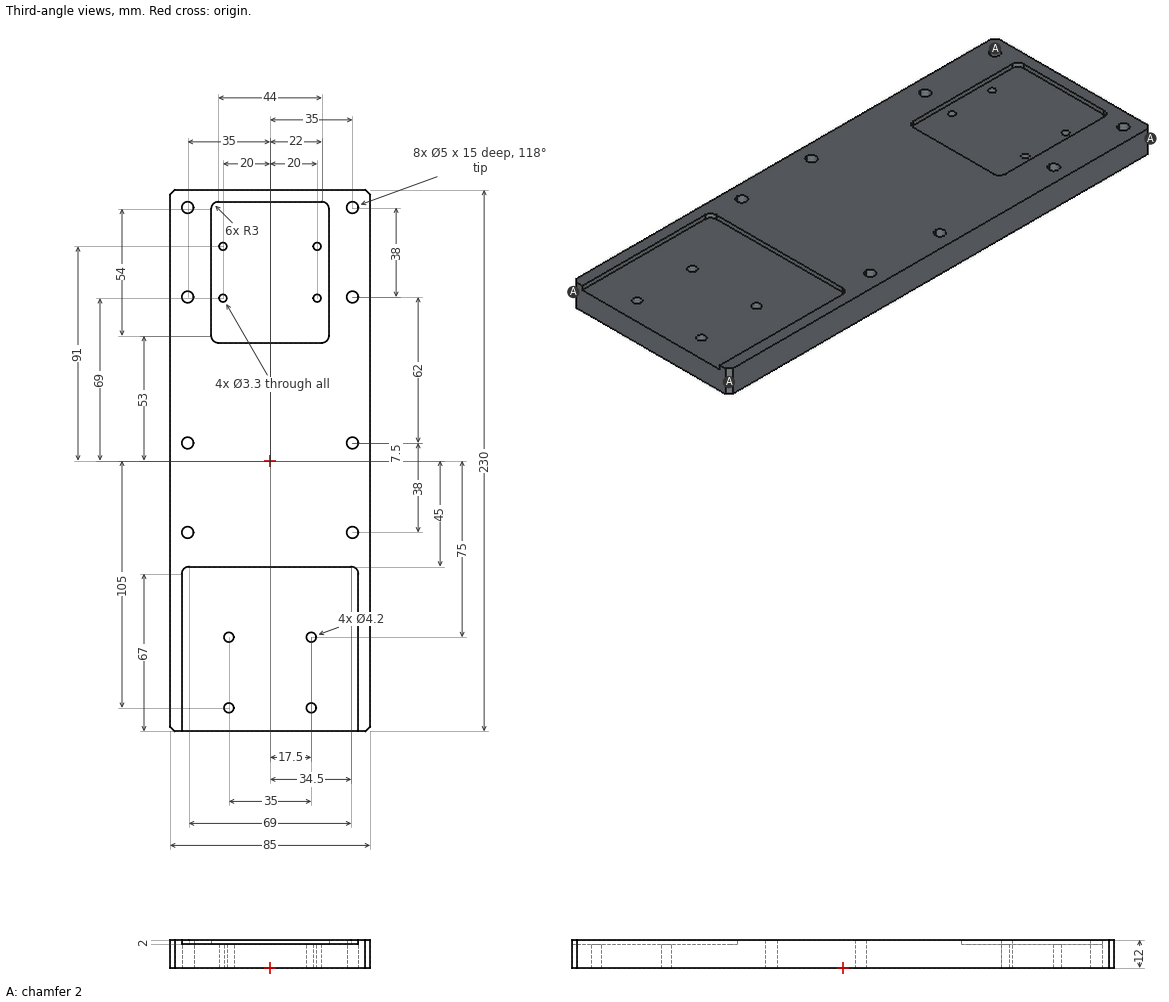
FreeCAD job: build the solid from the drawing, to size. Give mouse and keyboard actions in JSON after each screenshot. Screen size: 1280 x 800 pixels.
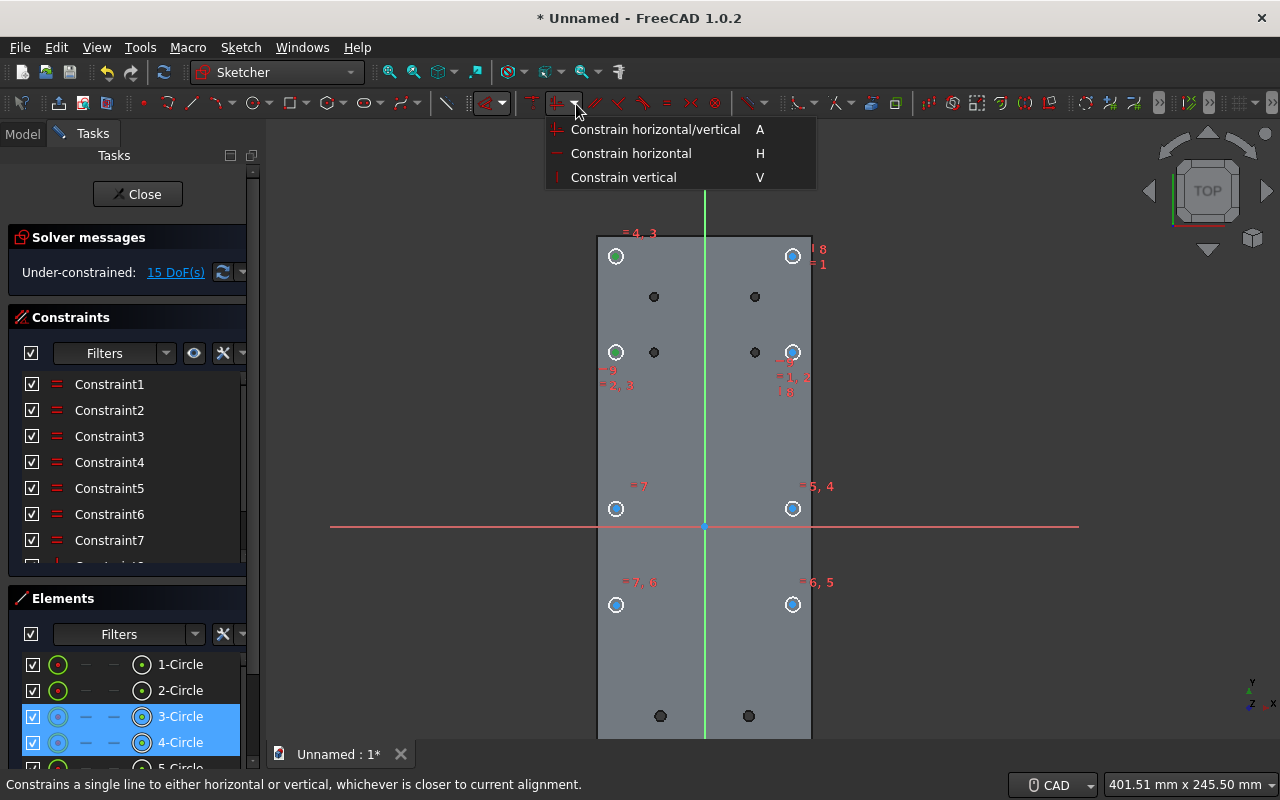
{"action": "left_click", "coordinate": [681, 177]}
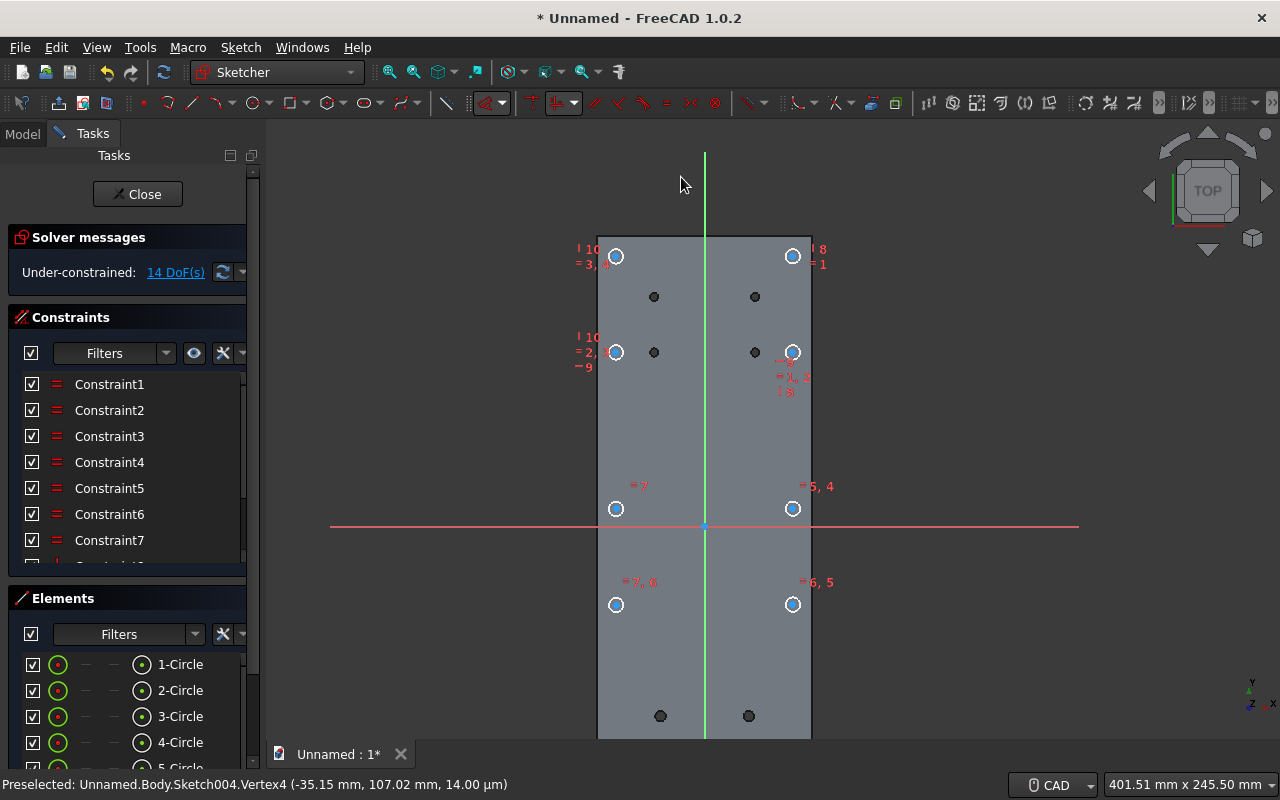
{"action": "left_click", "coordinate": [793, 256]}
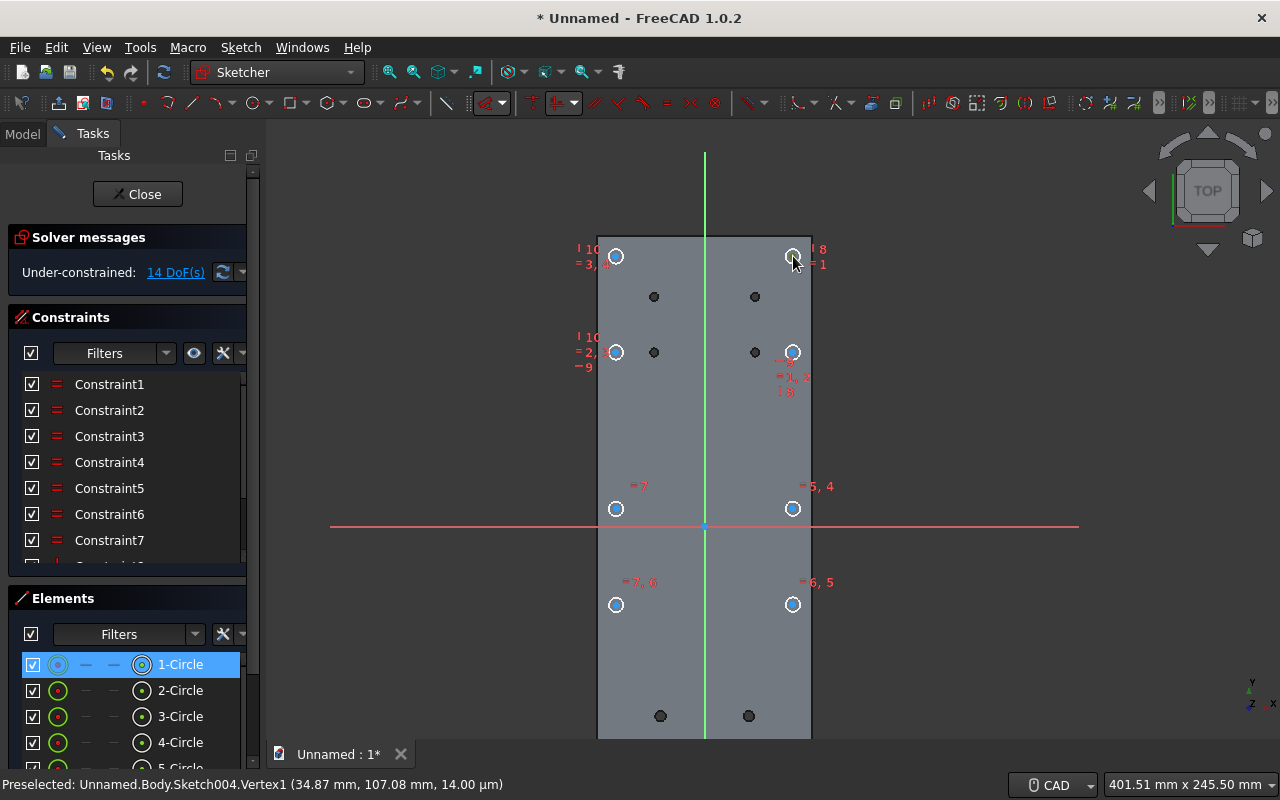
{"action": "left_click", "coordinate": [616, 256]}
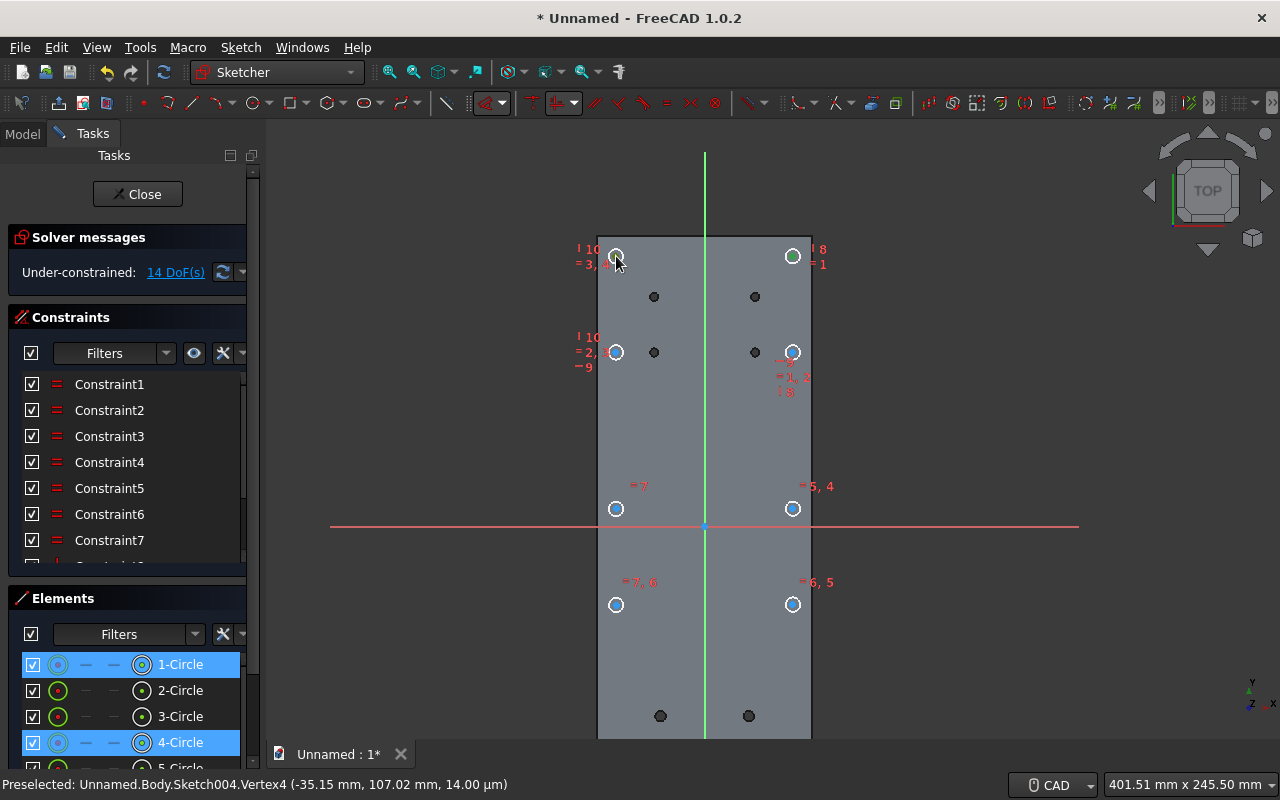
{"action": "key", "text": "h"}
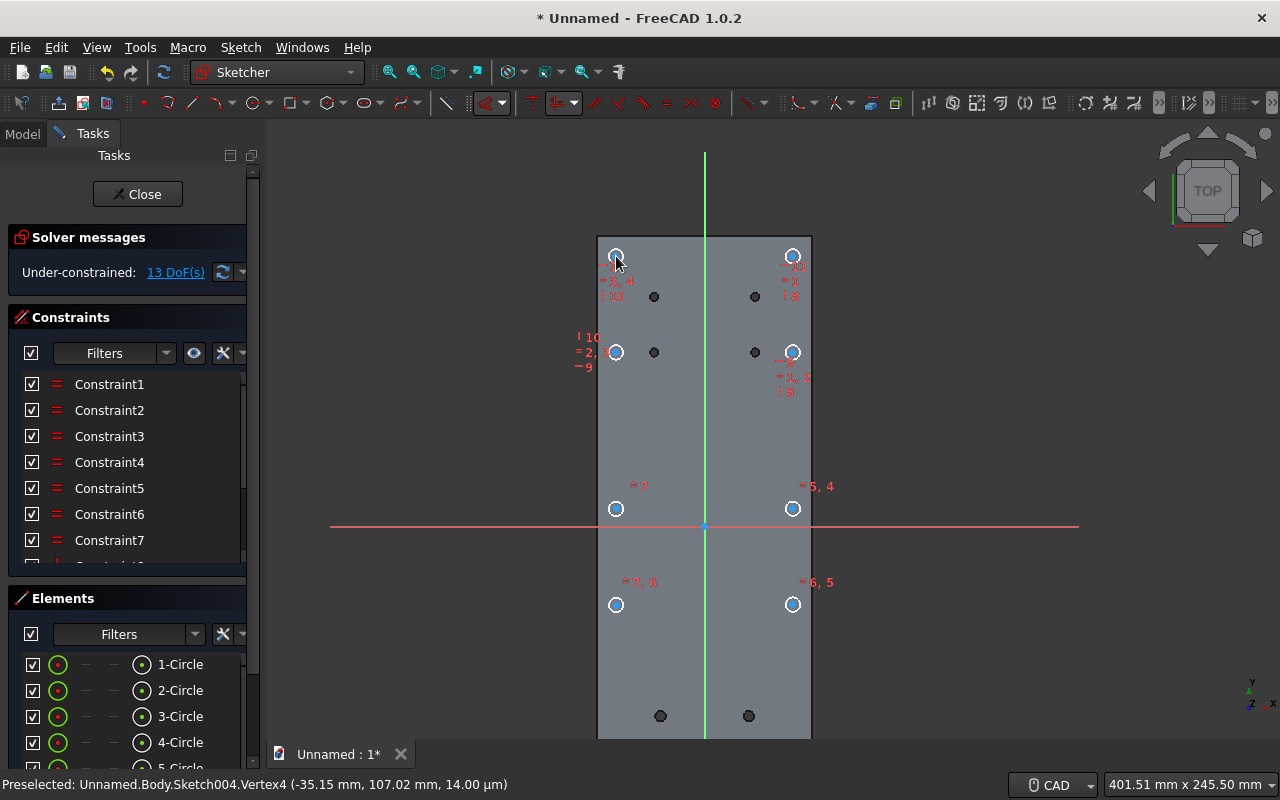
{"action": "left_click", "coordinate": [793, 352]}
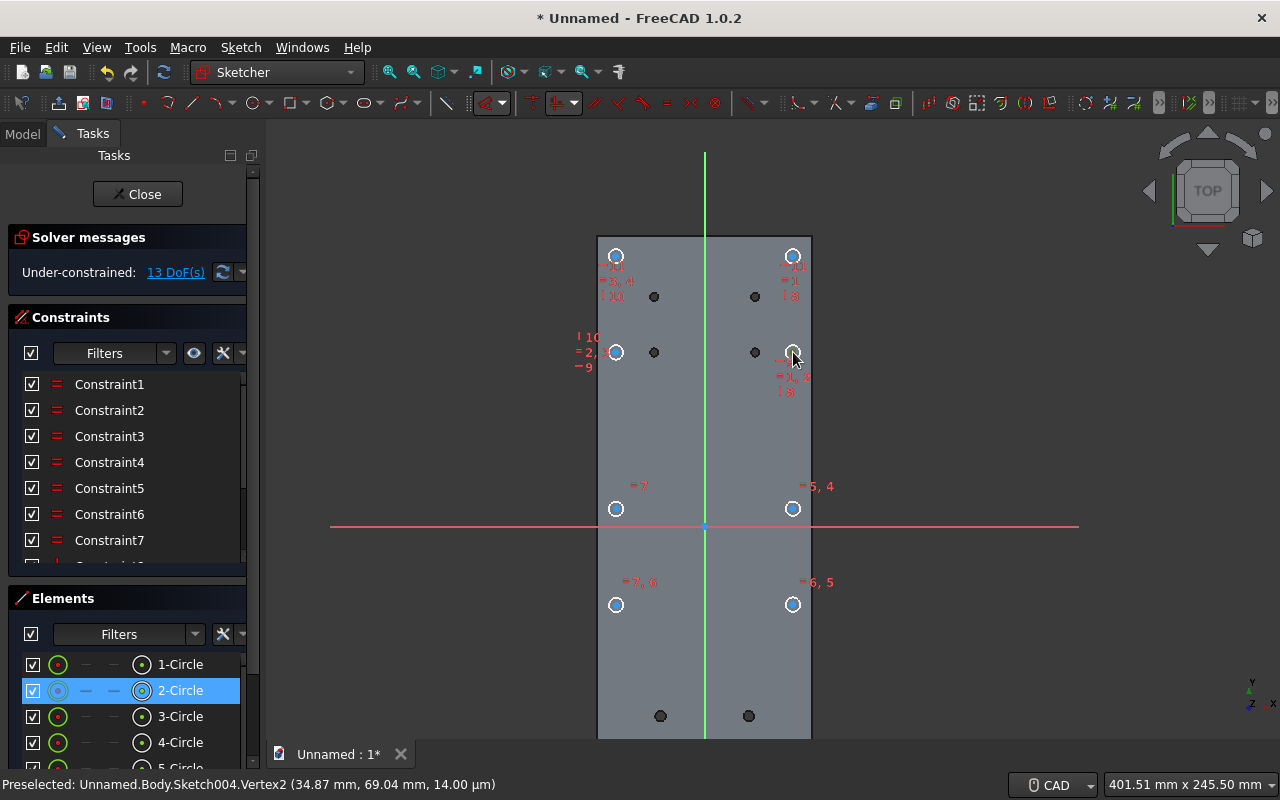
{"action": "left_click", "coordinate": [793, 509]}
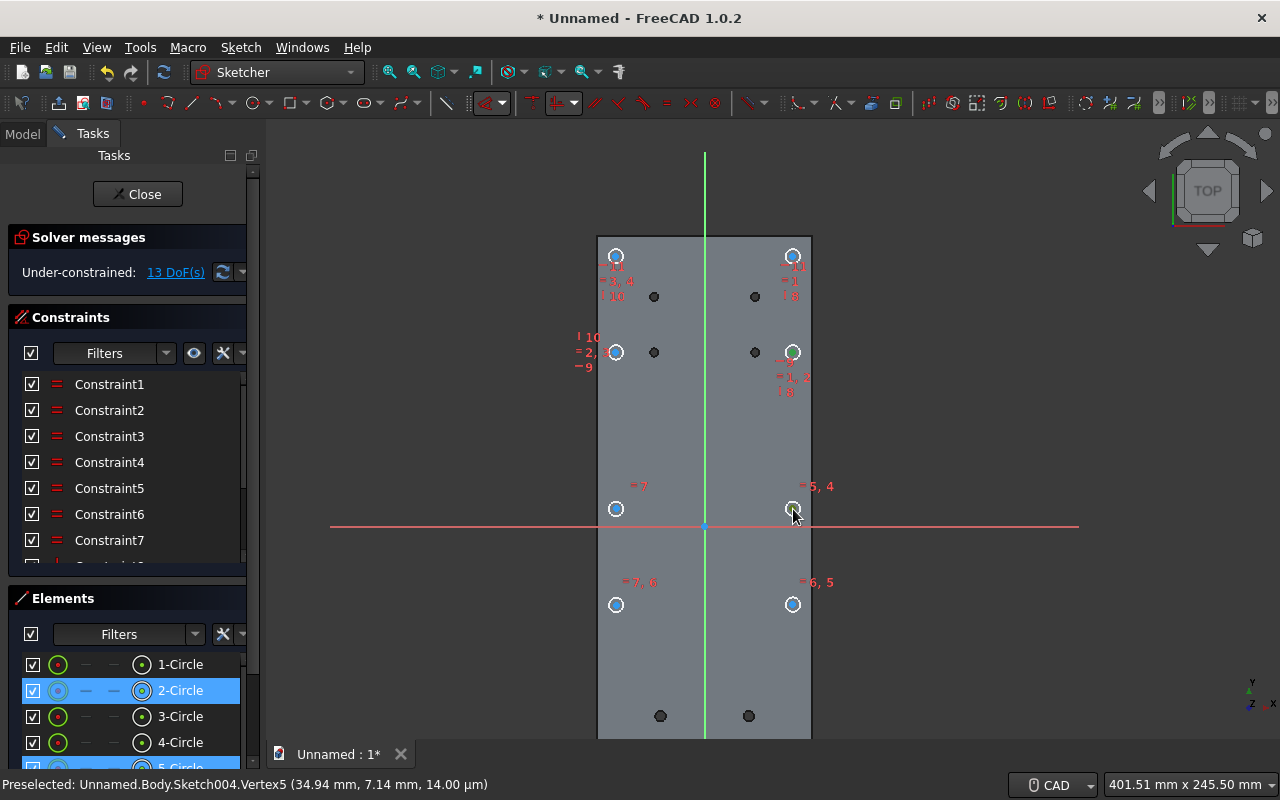
{"action": "key", "text": "v"}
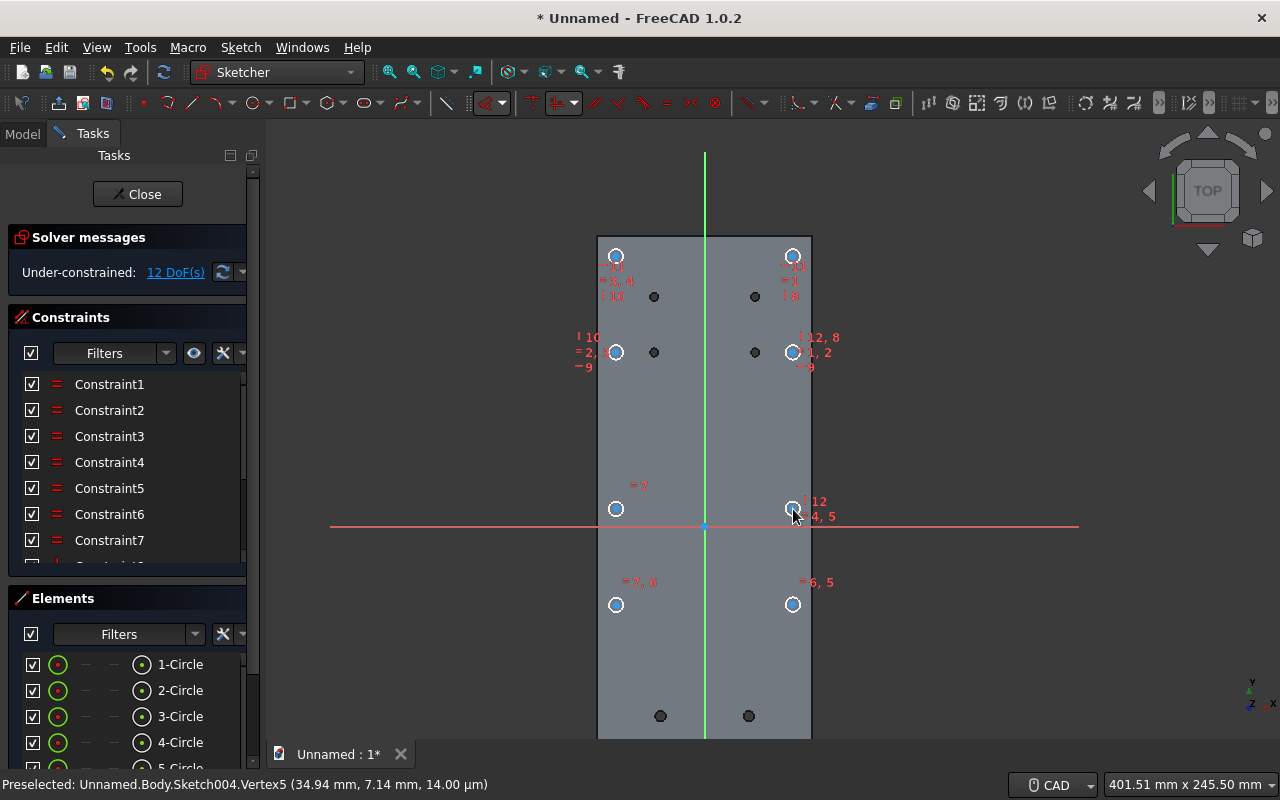
{"action": "left_click", "coordinate": [793, 509]}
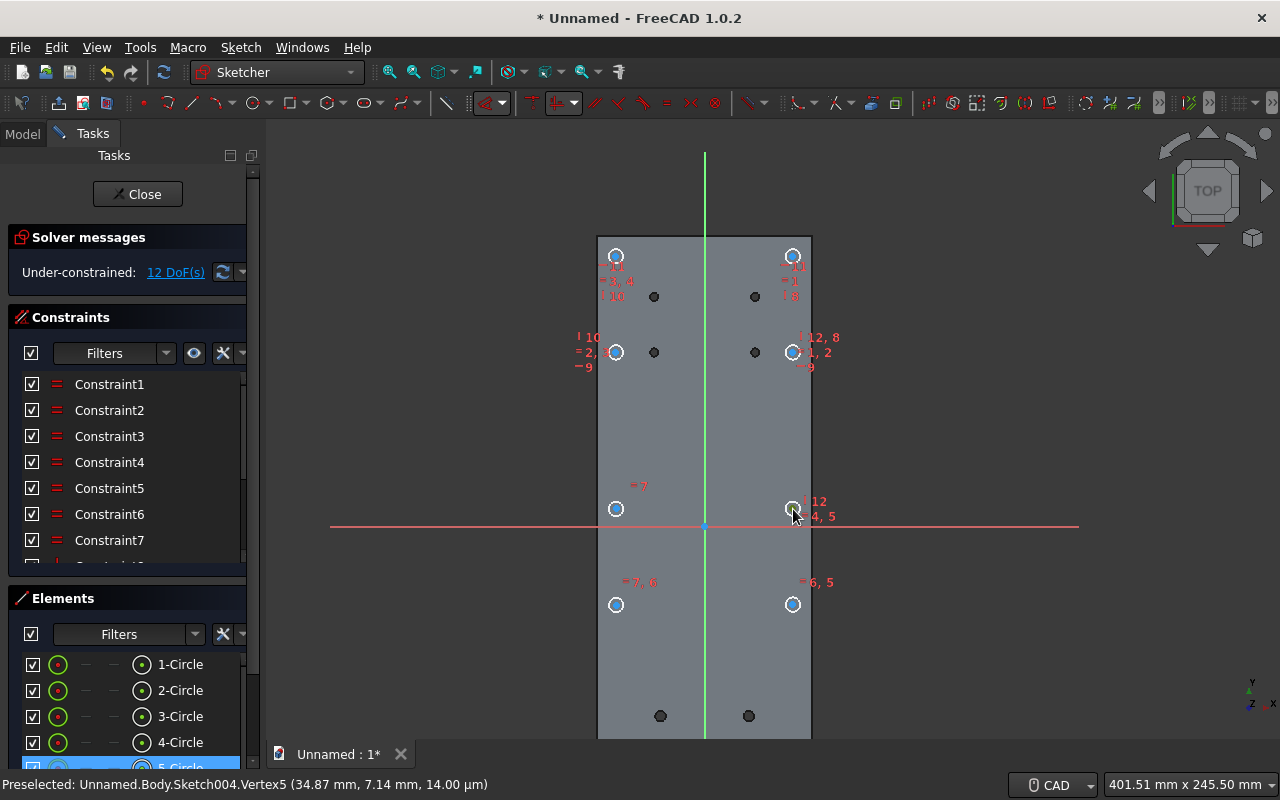
{"action": "left_click", "coordinate": [793, 605]}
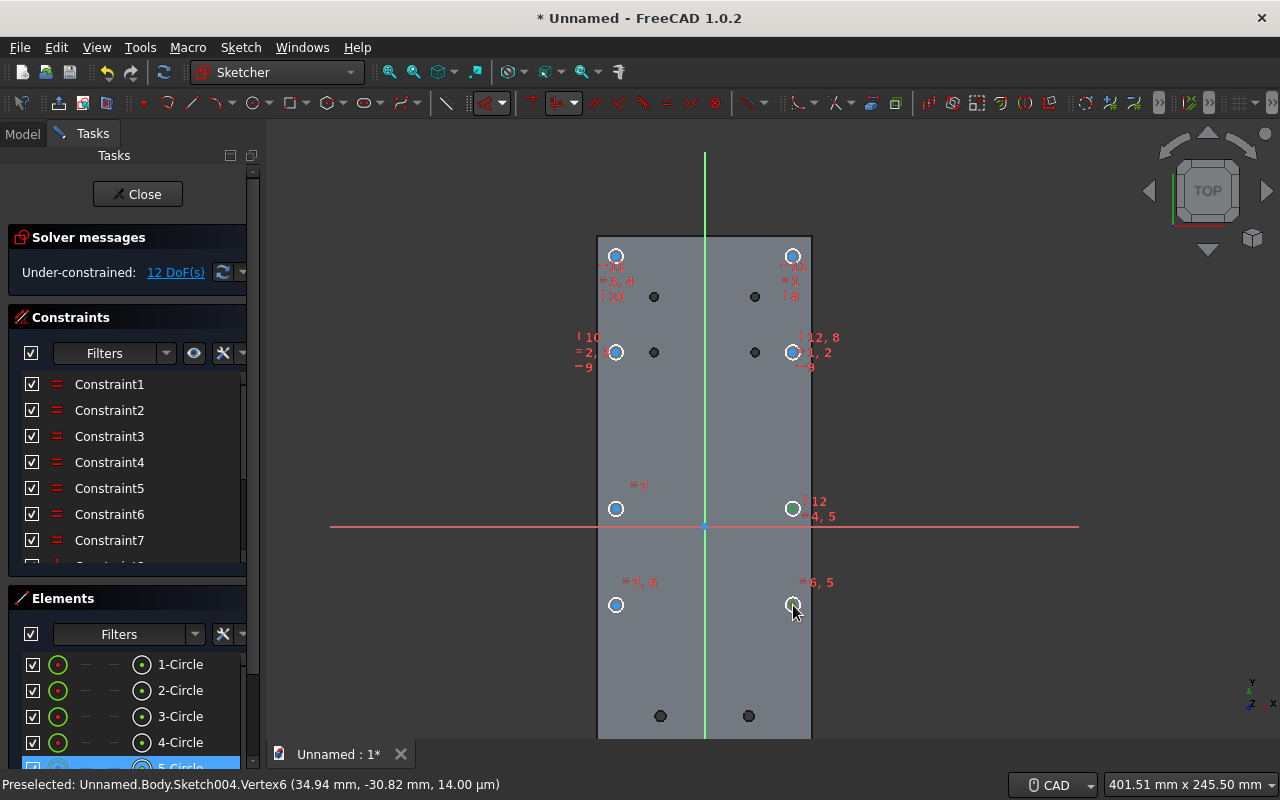
{"action": "left_click", "coordinate": [576, 104]}